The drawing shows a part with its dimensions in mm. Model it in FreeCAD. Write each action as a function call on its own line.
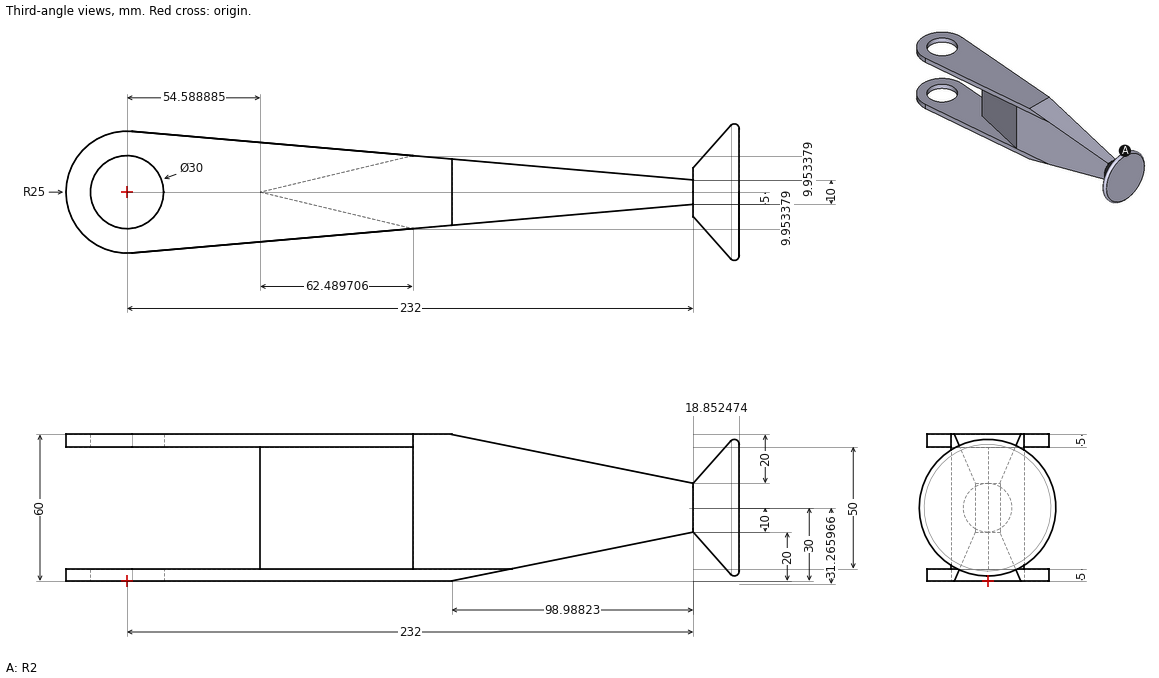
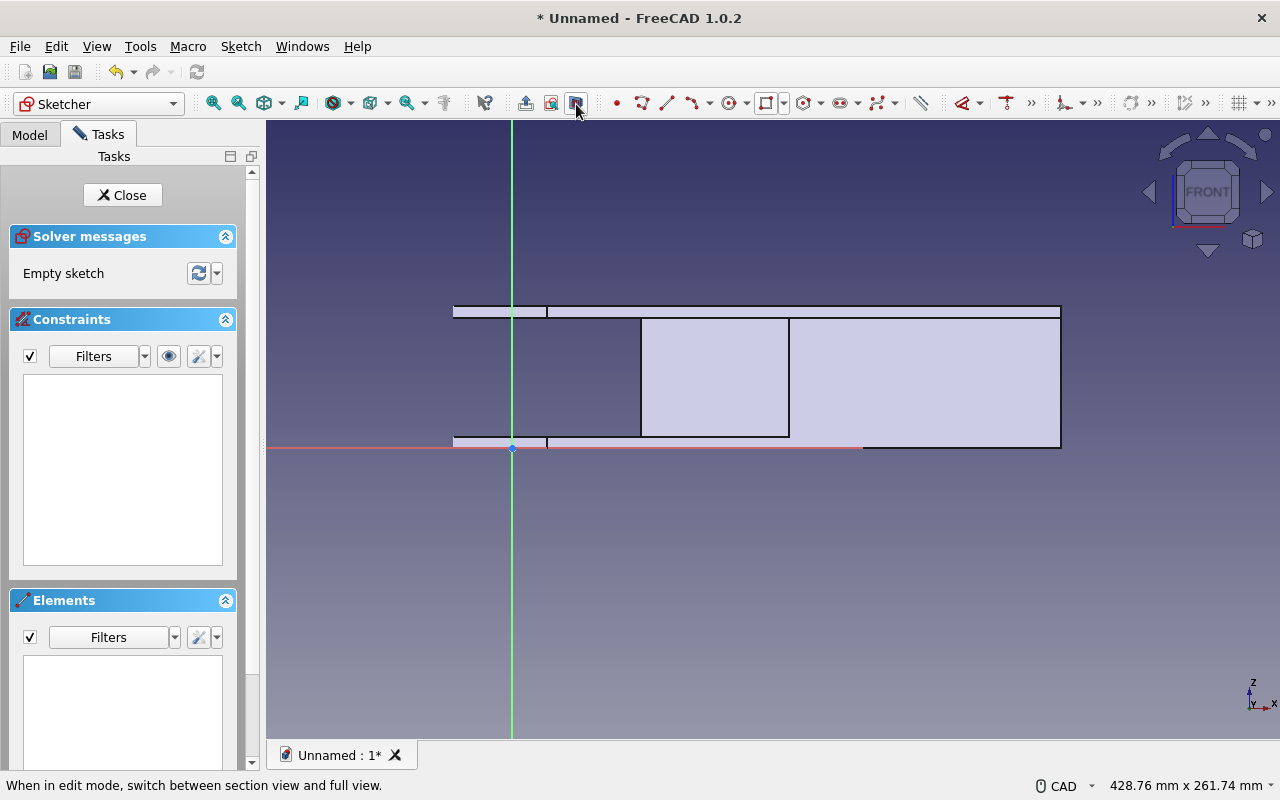
click(642, 104)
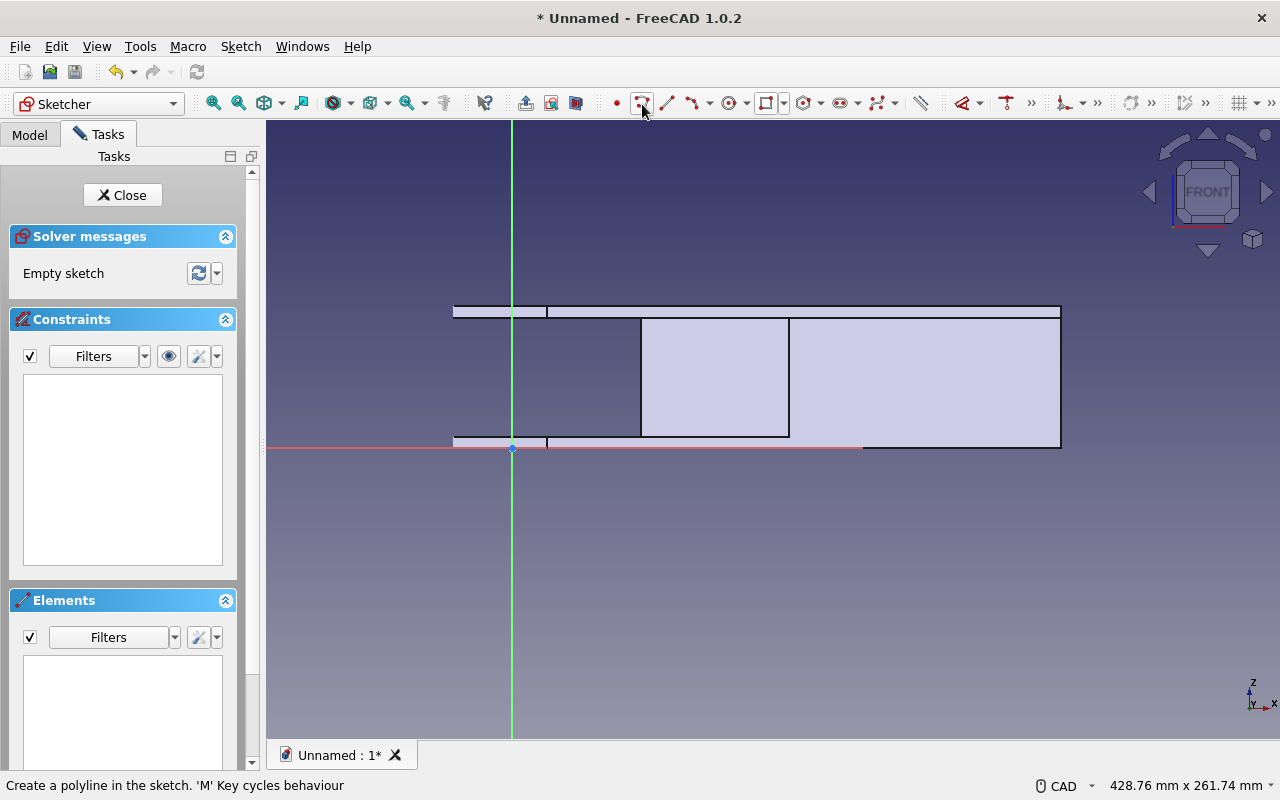
click(827, 448)
click(1061, 401)
click(1061, 439)
click(827, 448)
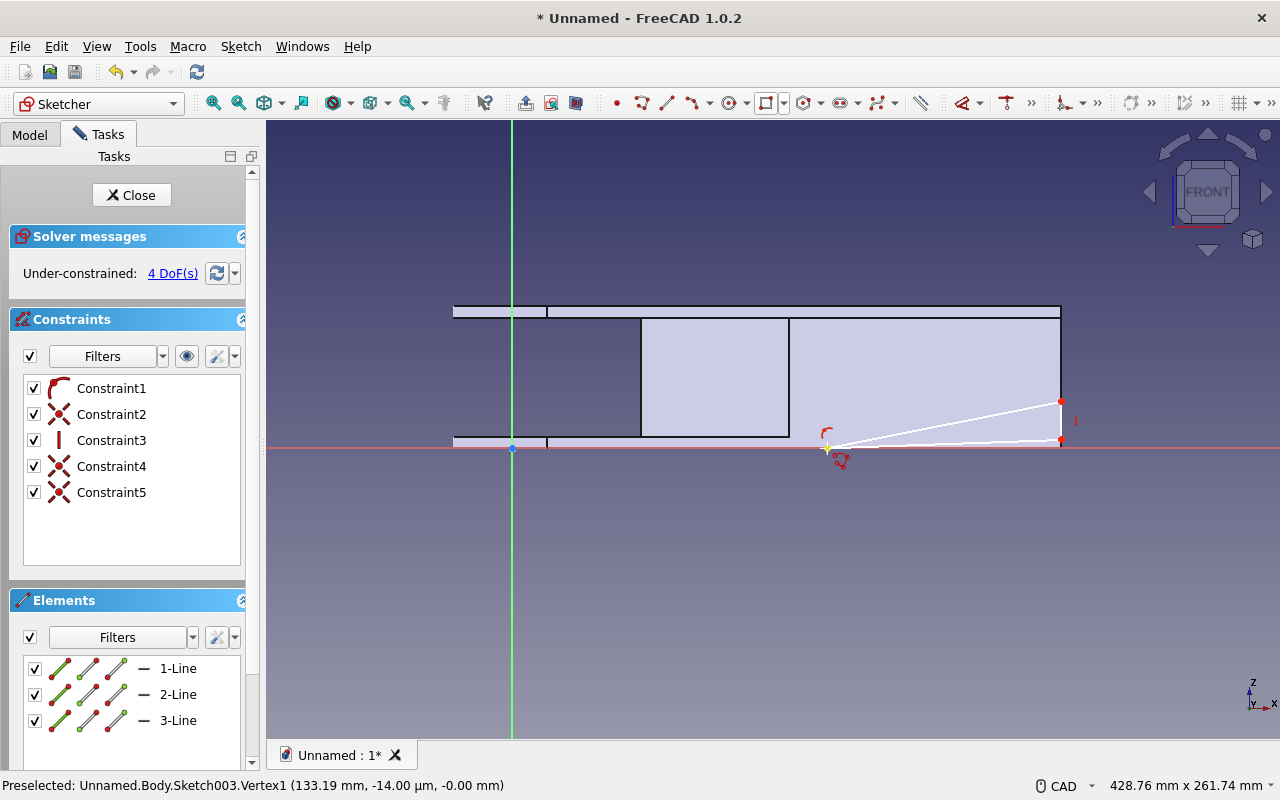
click(827, 306)
click(1061, 306)
click(1061, 354)
click(827, 307)
key(Escape)
key(Escape)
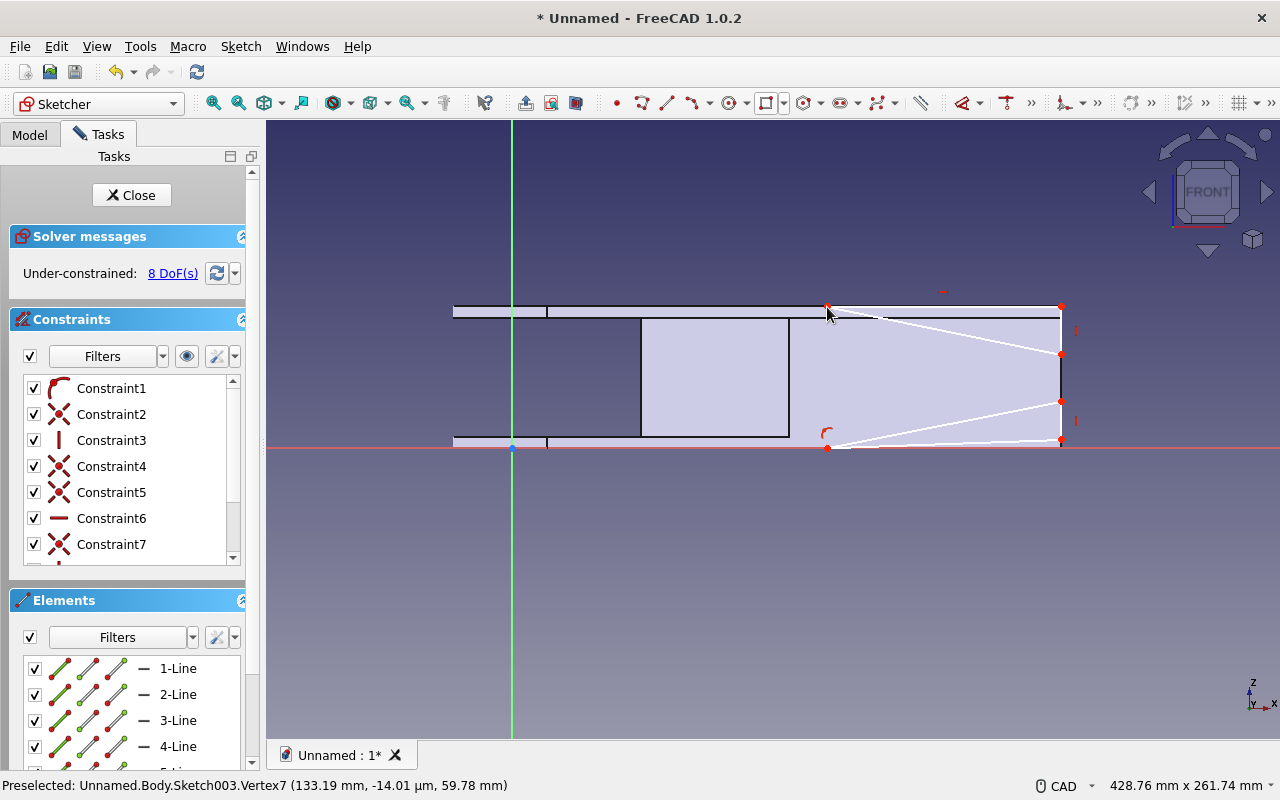
scroll(897, 446, up, 2)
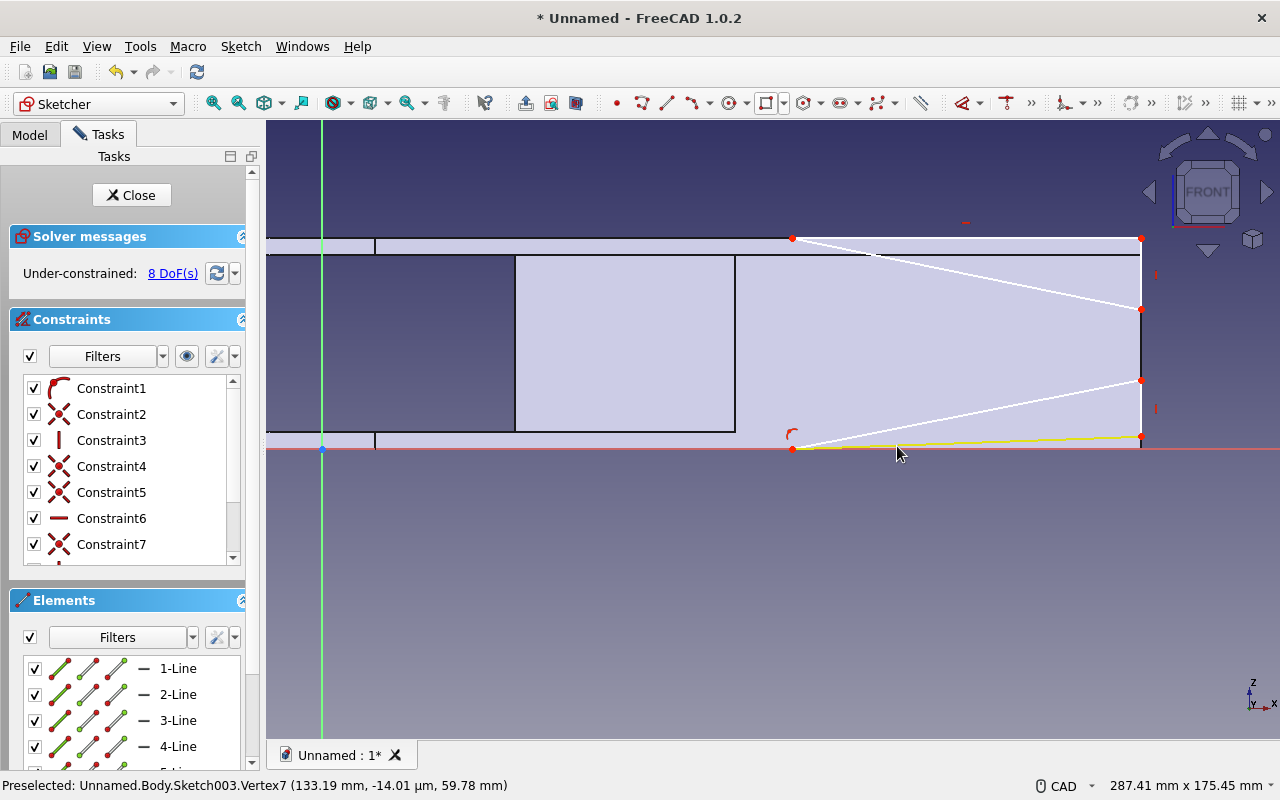
click(897, 446)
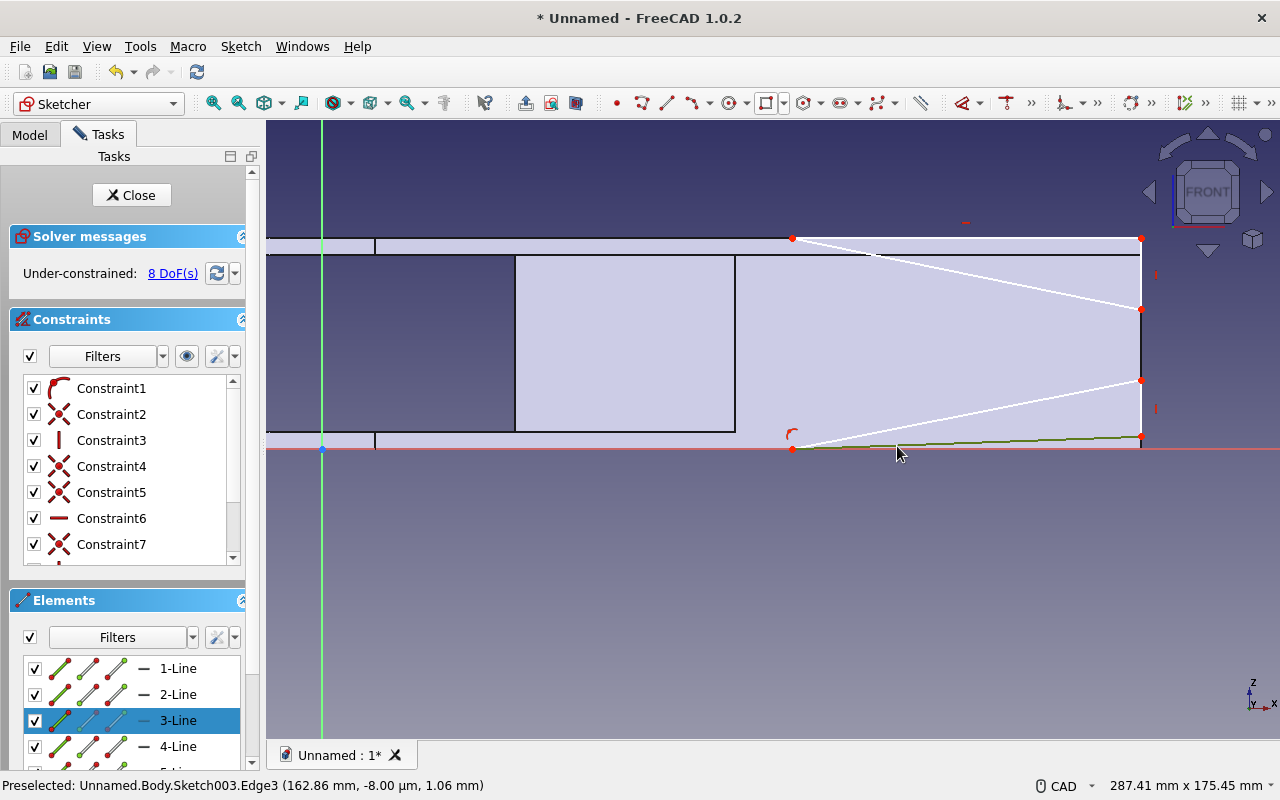
key(h)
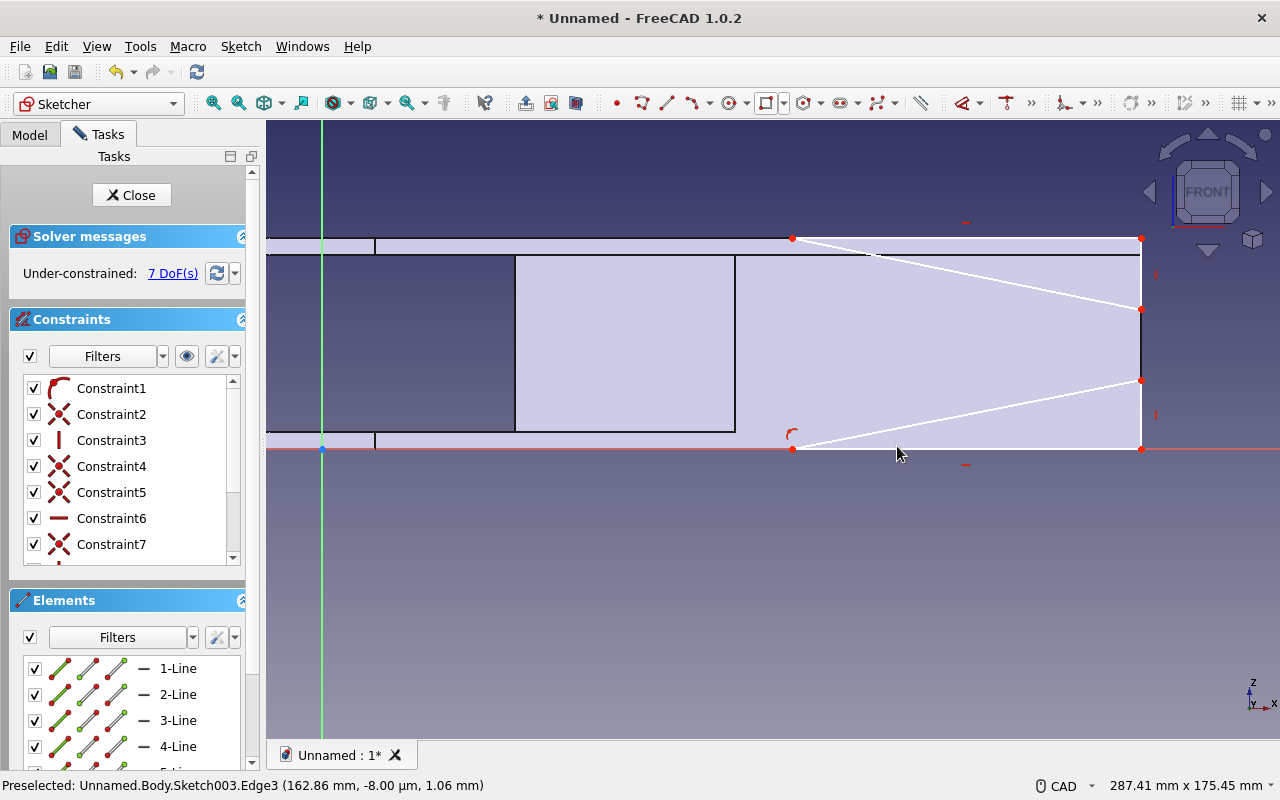
click(962, 104)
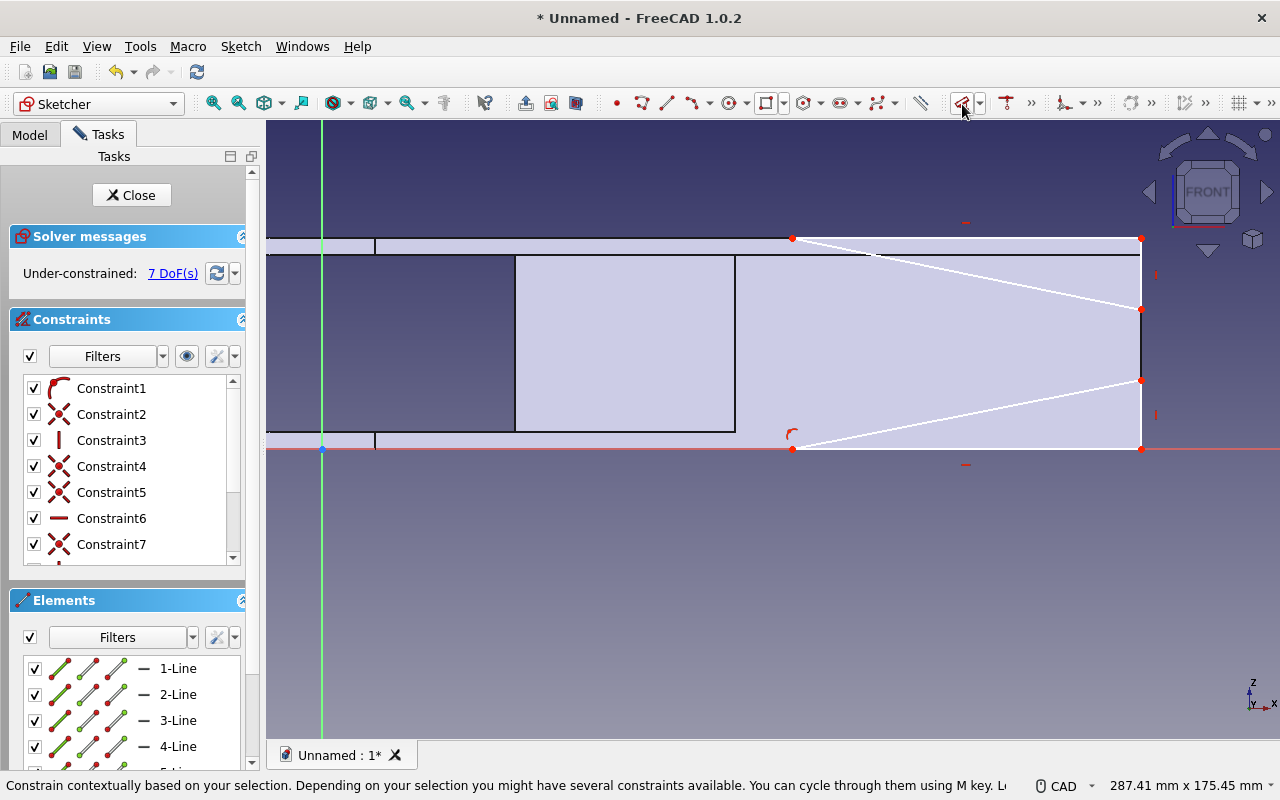
scroll(649, 604, down, 2)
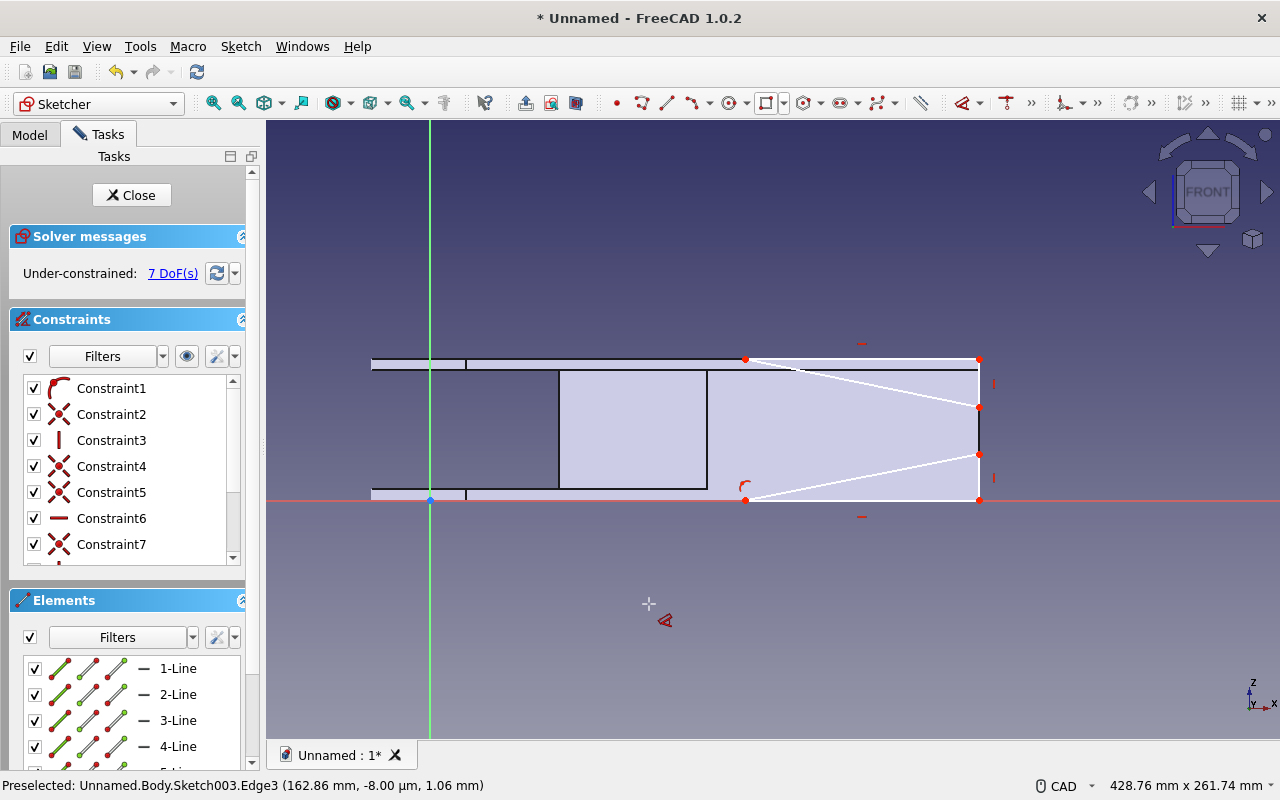
click(979, 468)
click(1013, 477)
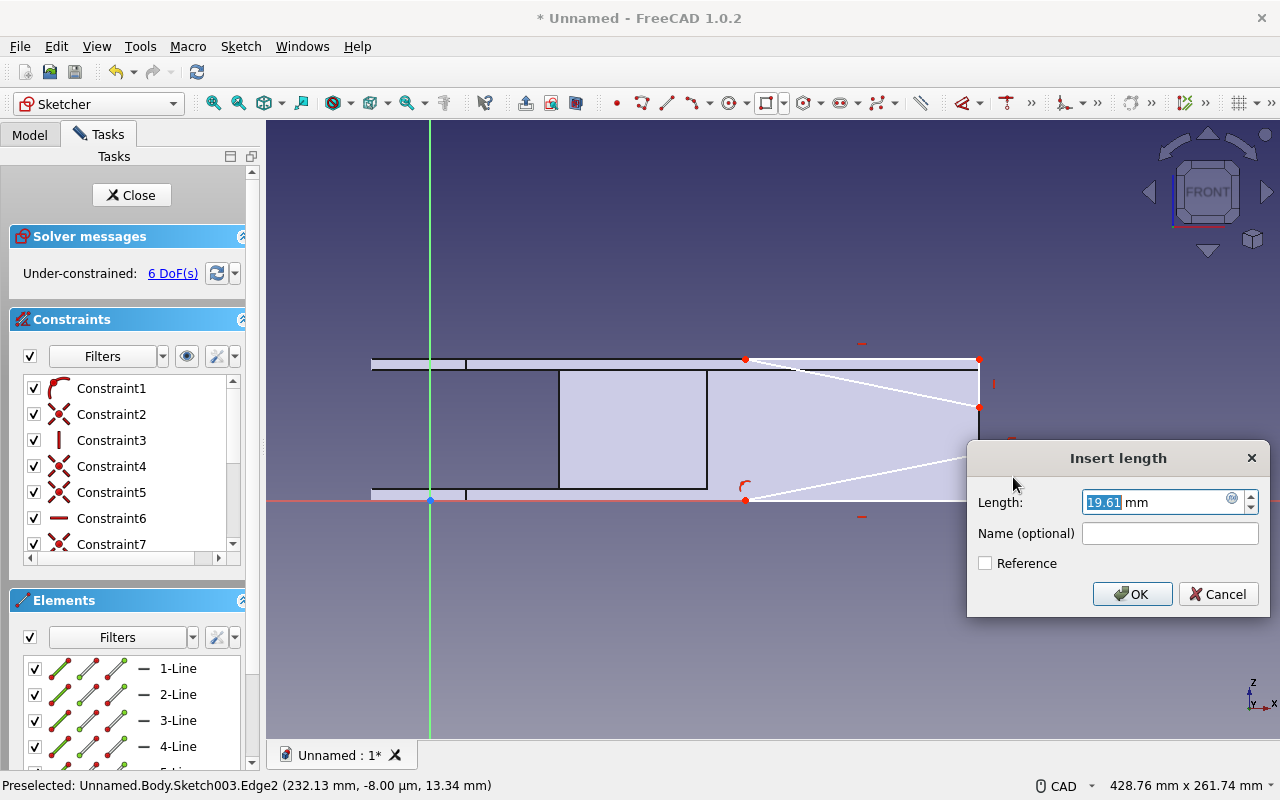
text(20)
key(Return)